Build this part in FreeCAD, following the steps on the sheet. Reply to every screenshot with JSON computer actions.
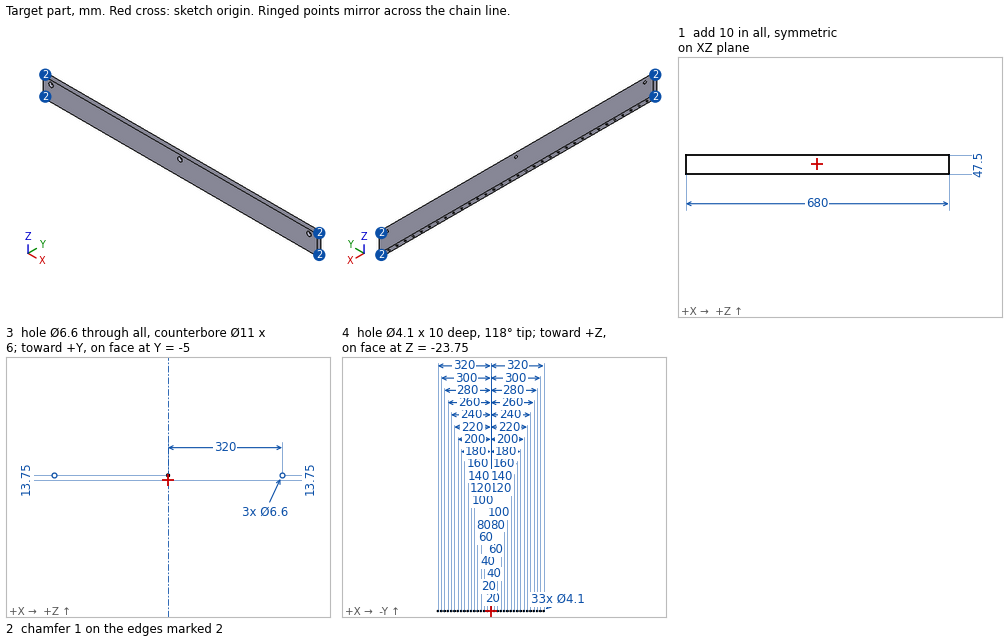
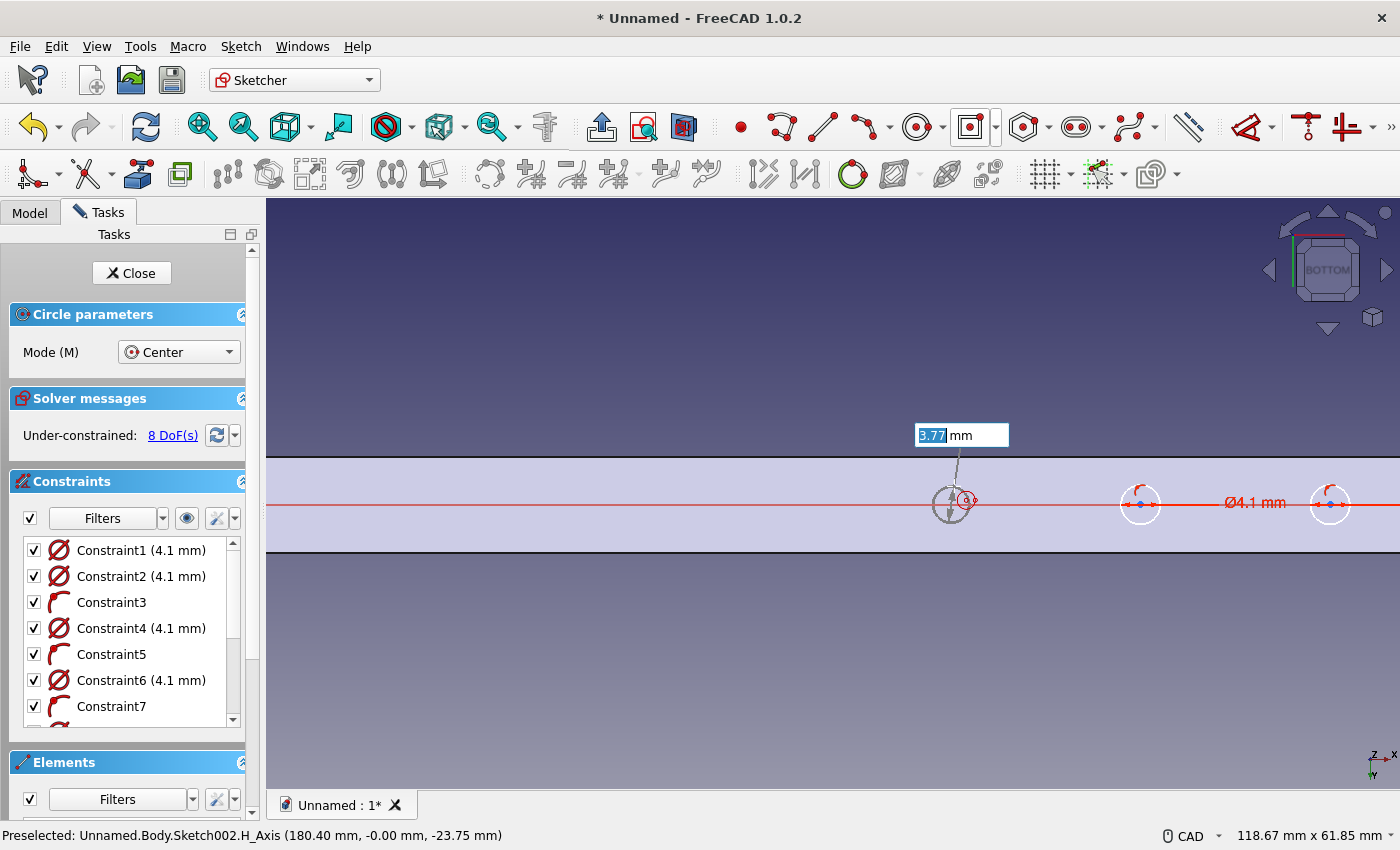
{"action": "type", "text": "4.1"}
{"action": "key", "text": "Return"}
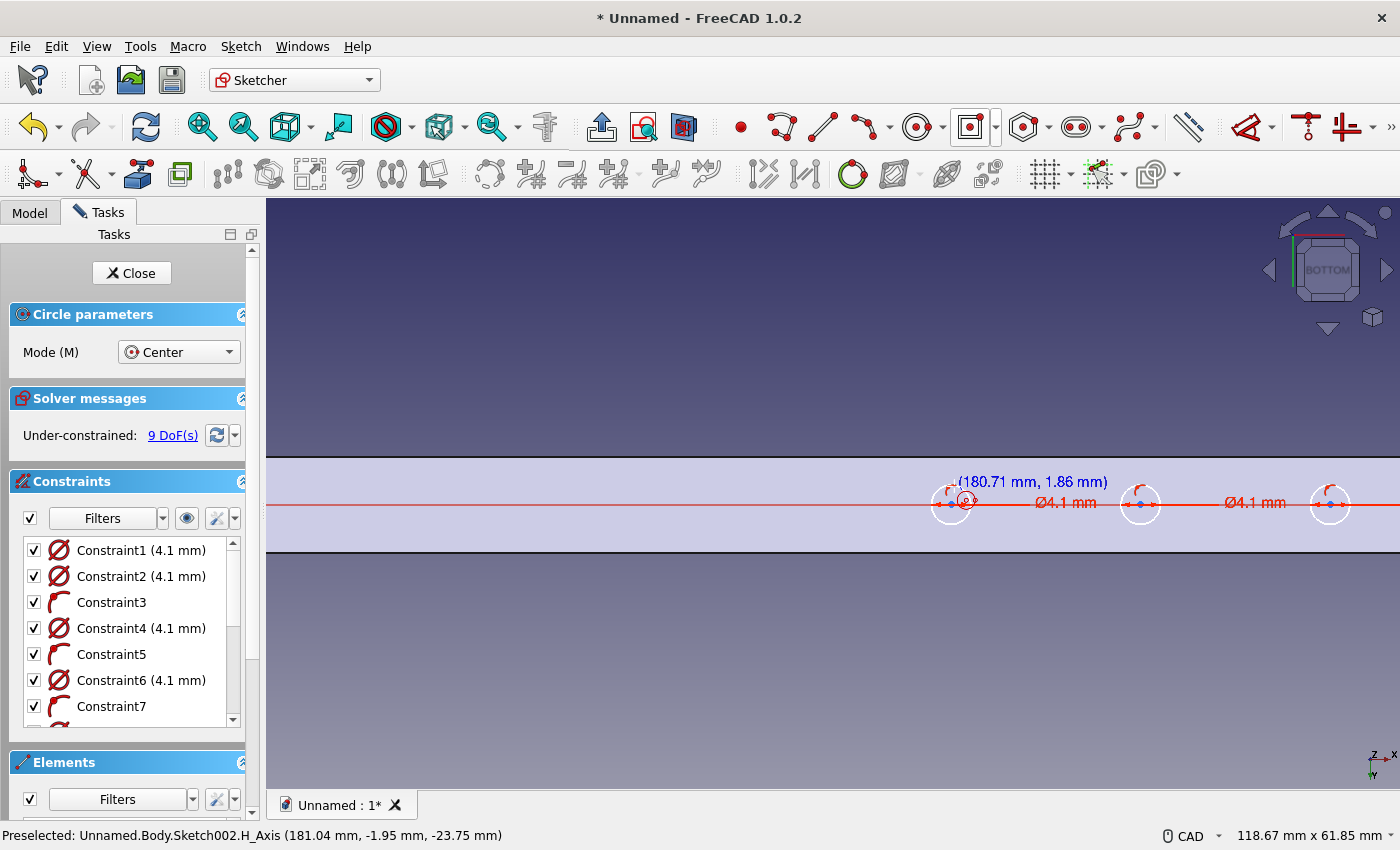
{"action": "scroll", "coordinate": [956, 492], "scroll_direction": "down", "scroll_amount": 11}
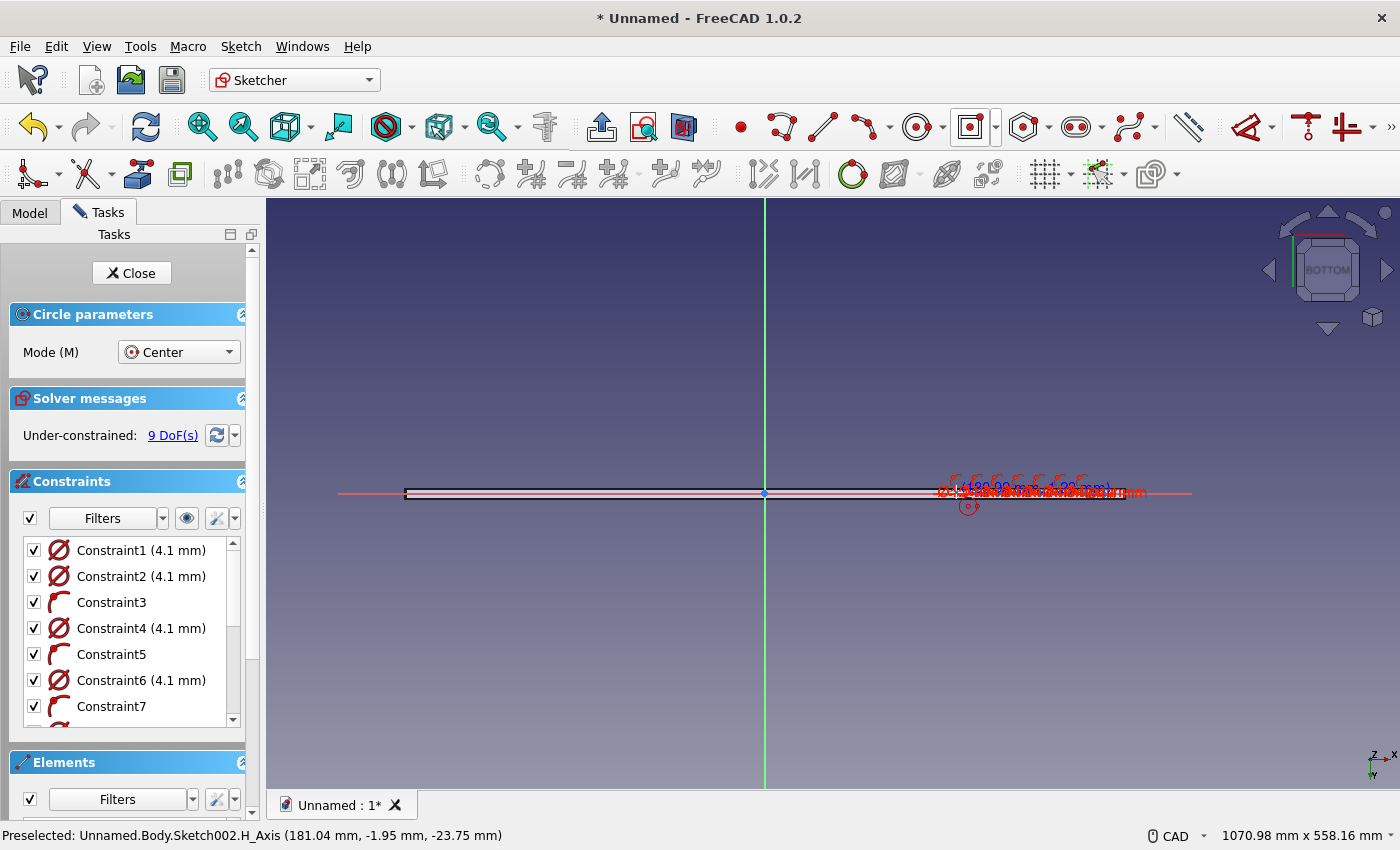
{"action": "left_click", "coordinate": [934, 494]}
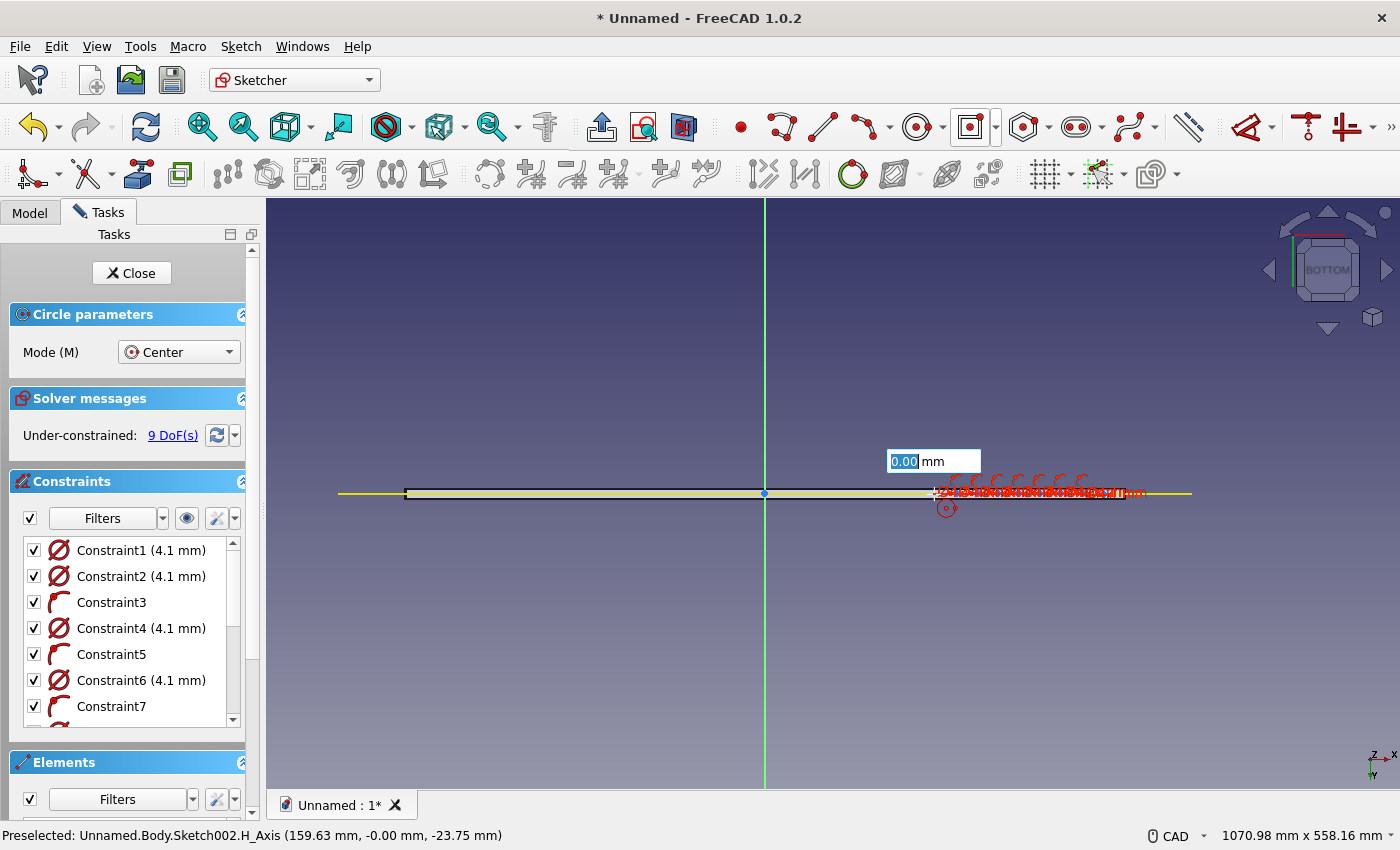
{"action": "scroll", "coordinate": [935, 492], "scroll_direction": "up", "scroll_amount": 11}
{"action": "mouse_move", "coordinate": [931, 486]}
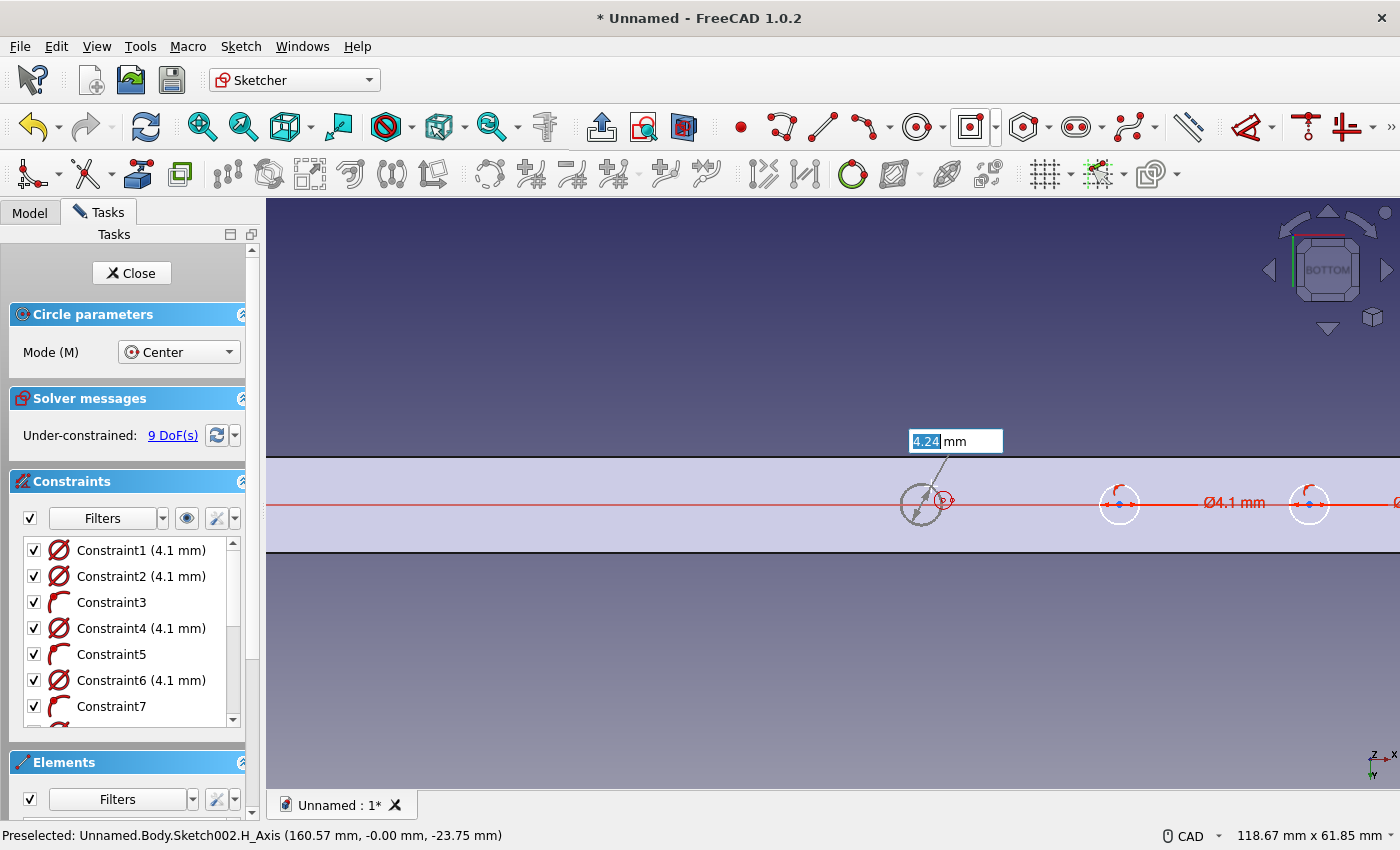
{"action": "type", "text": "4.1"}
{"action": "key", "text": "Return"}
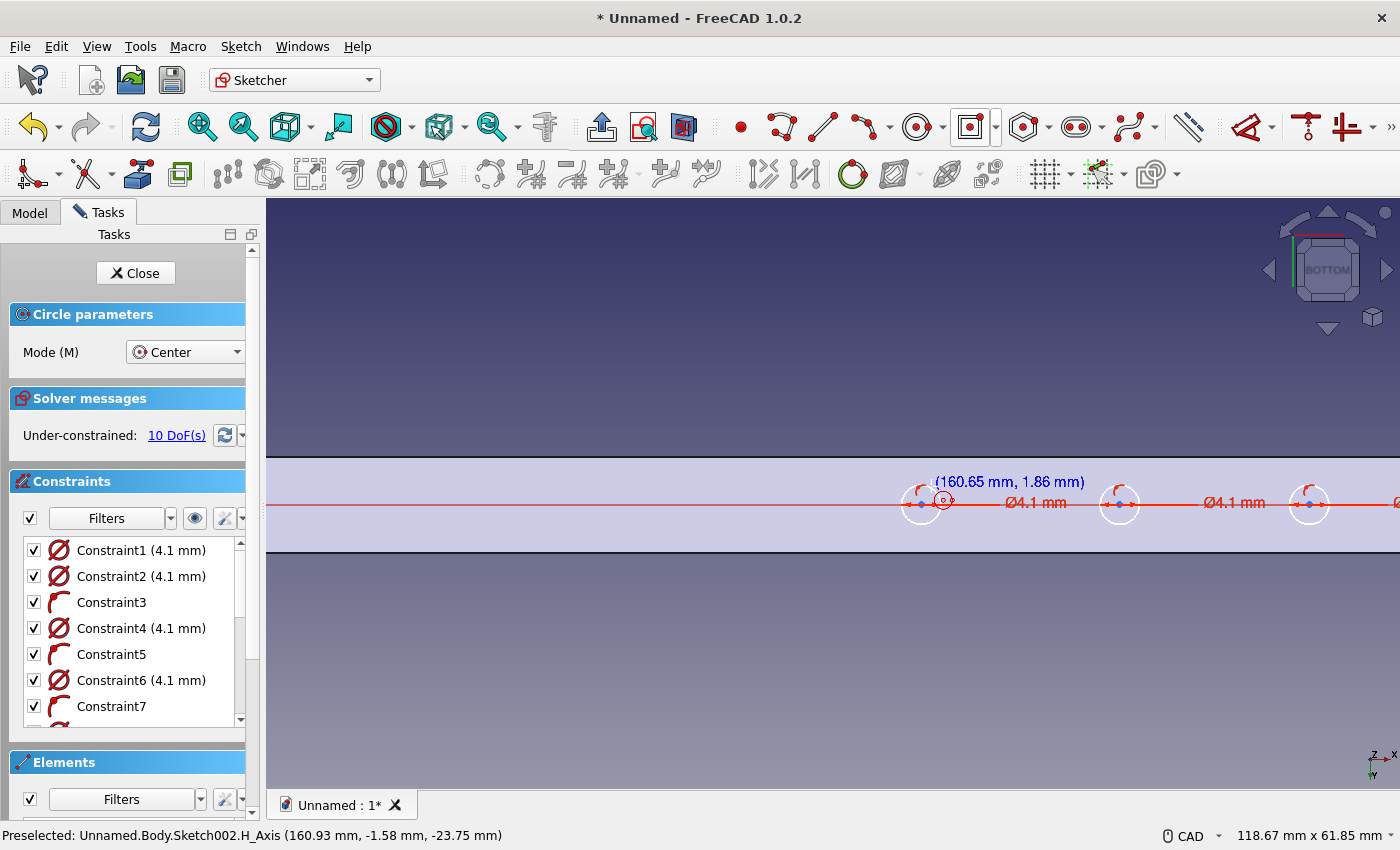
{"action": "scroll", "coordinate": [935, 492], "scroll_direction": "down", "scroll_amount": 11}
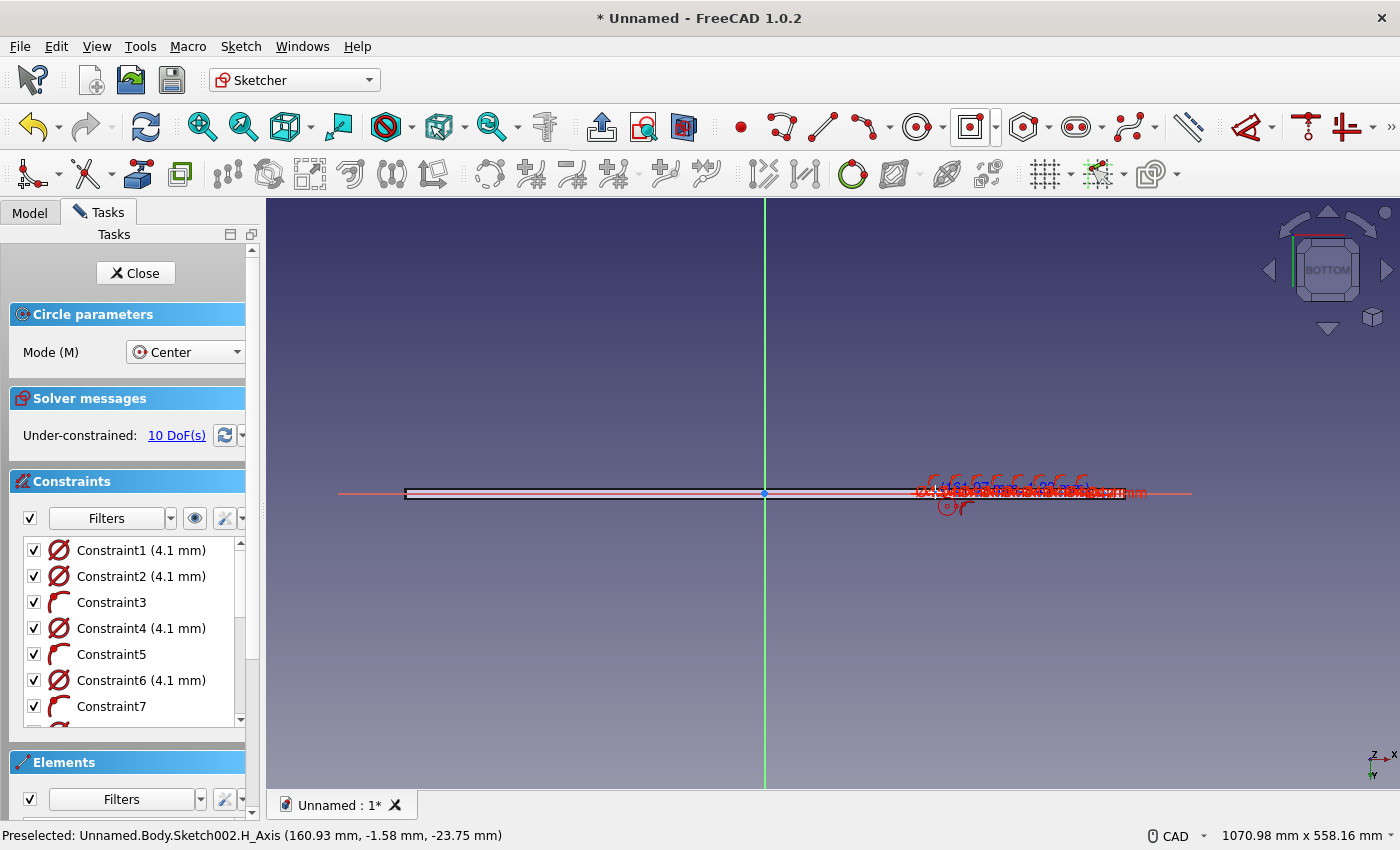
{"action": "left_click", "coordinate": [913, 494]}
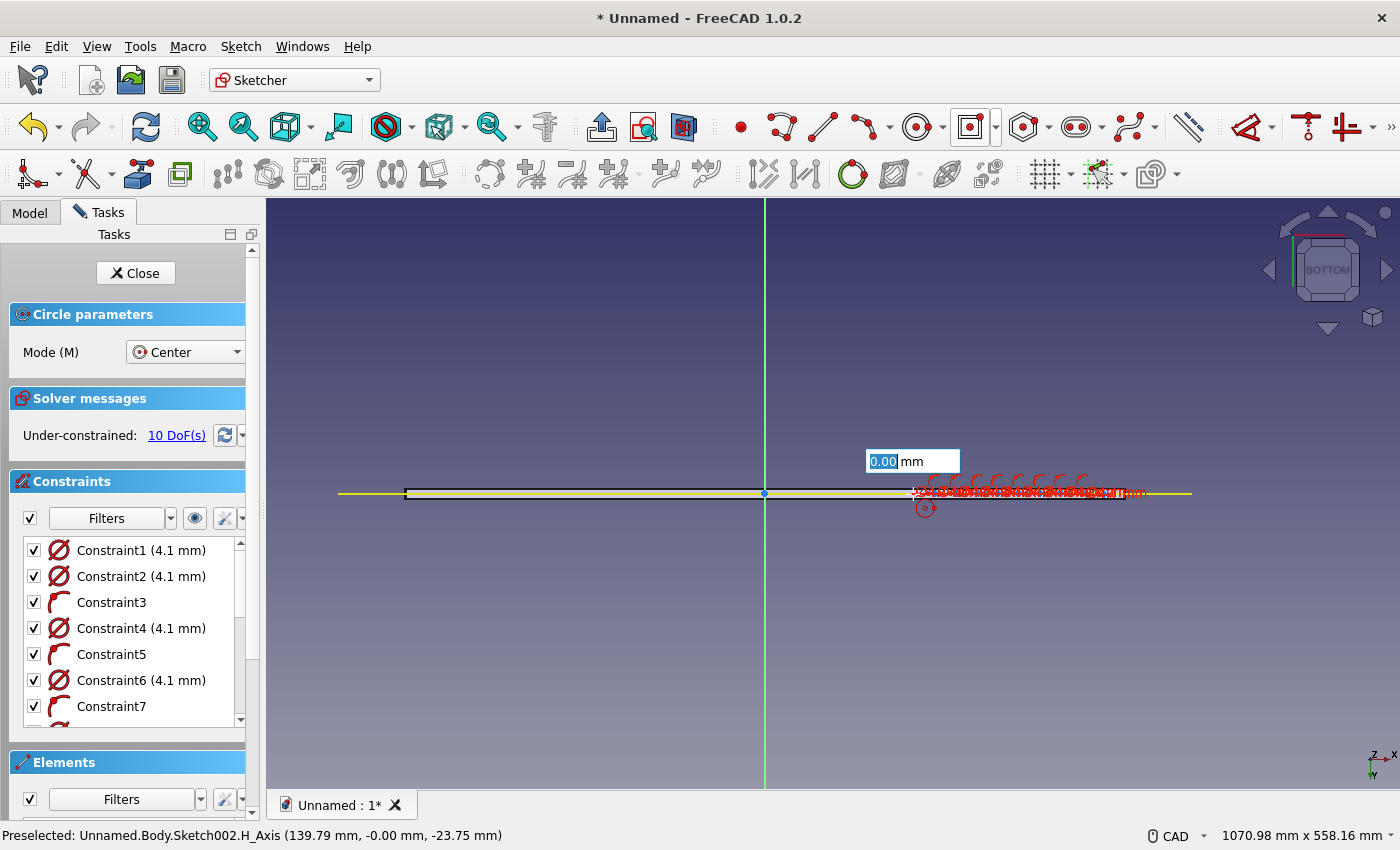
{"action": "scroll", "coordinate": [912, 496], "scroll_direction": "up", "scroll_amount": 11}
{"action": "mouse_move", "coordinate": [912, 491]}